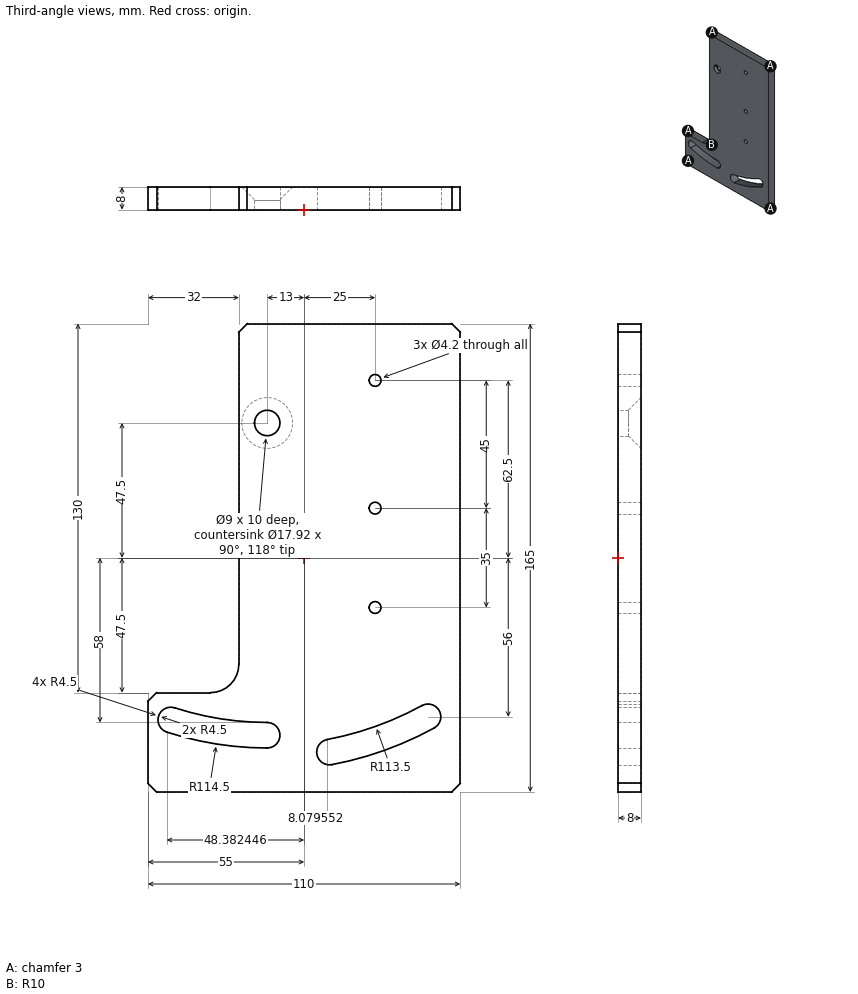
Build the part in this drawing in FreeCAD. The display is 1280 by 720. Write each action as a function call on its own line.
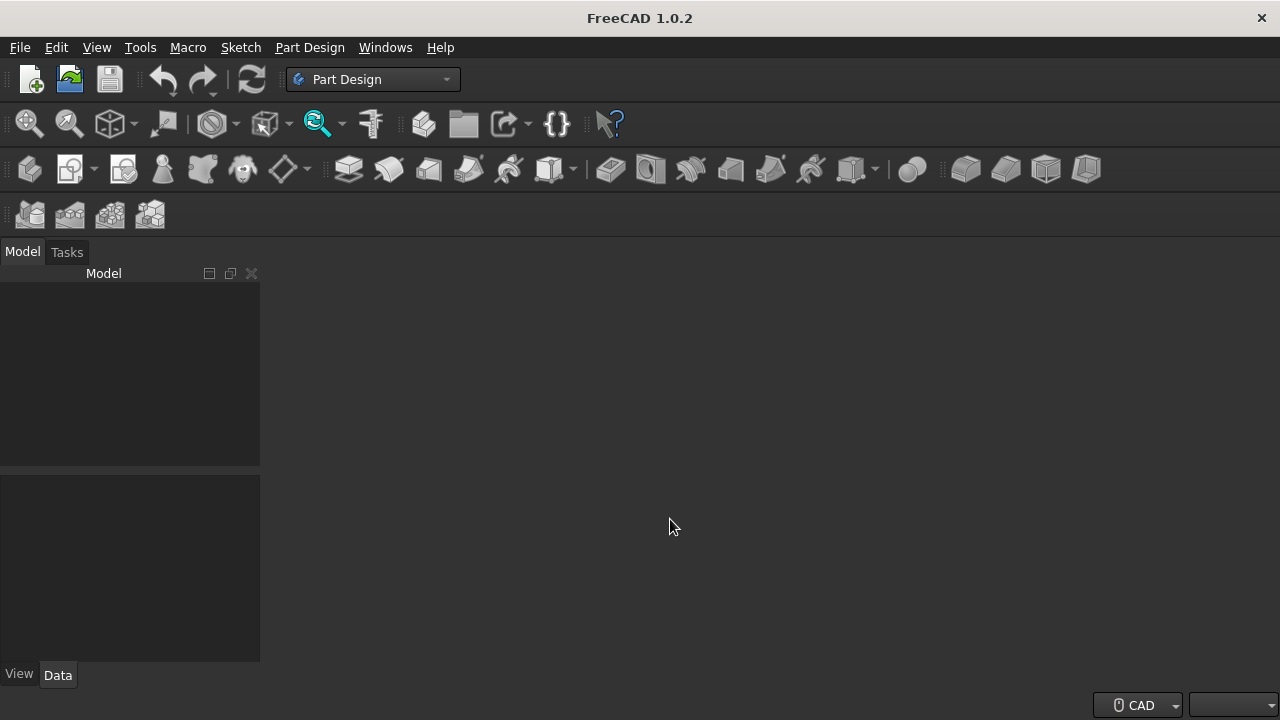
click(30, 80)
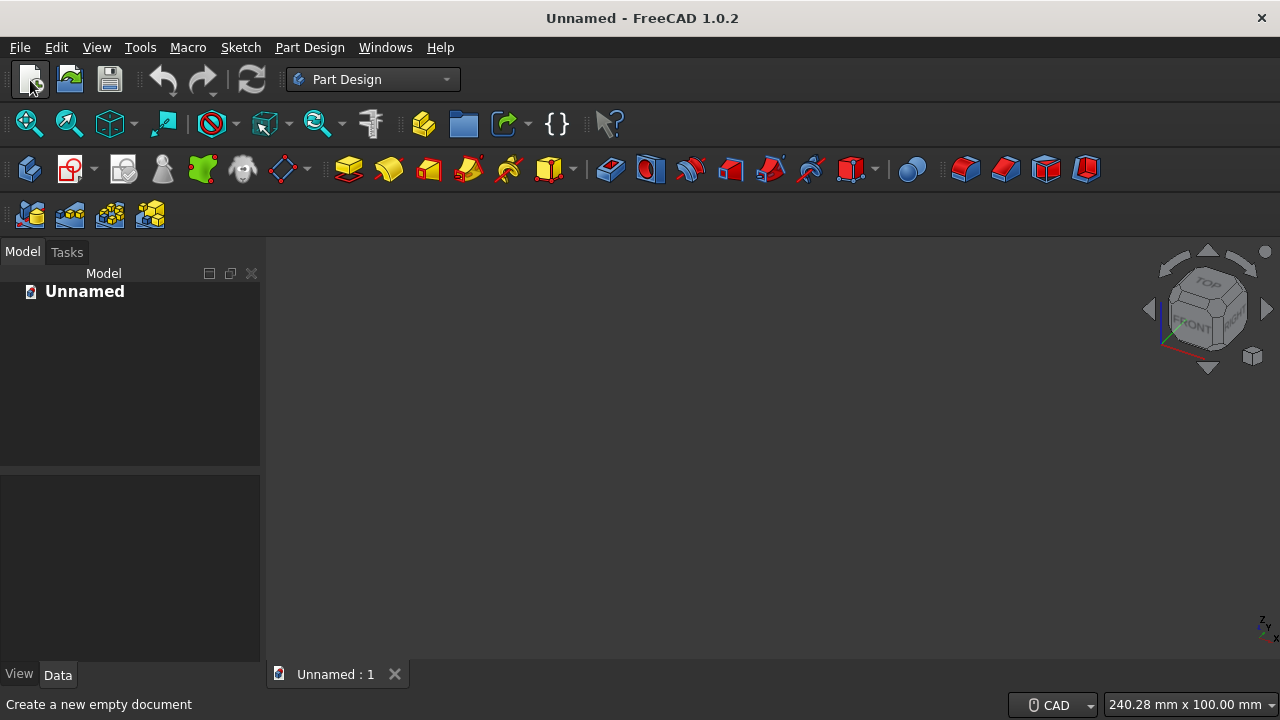
click(70, 170)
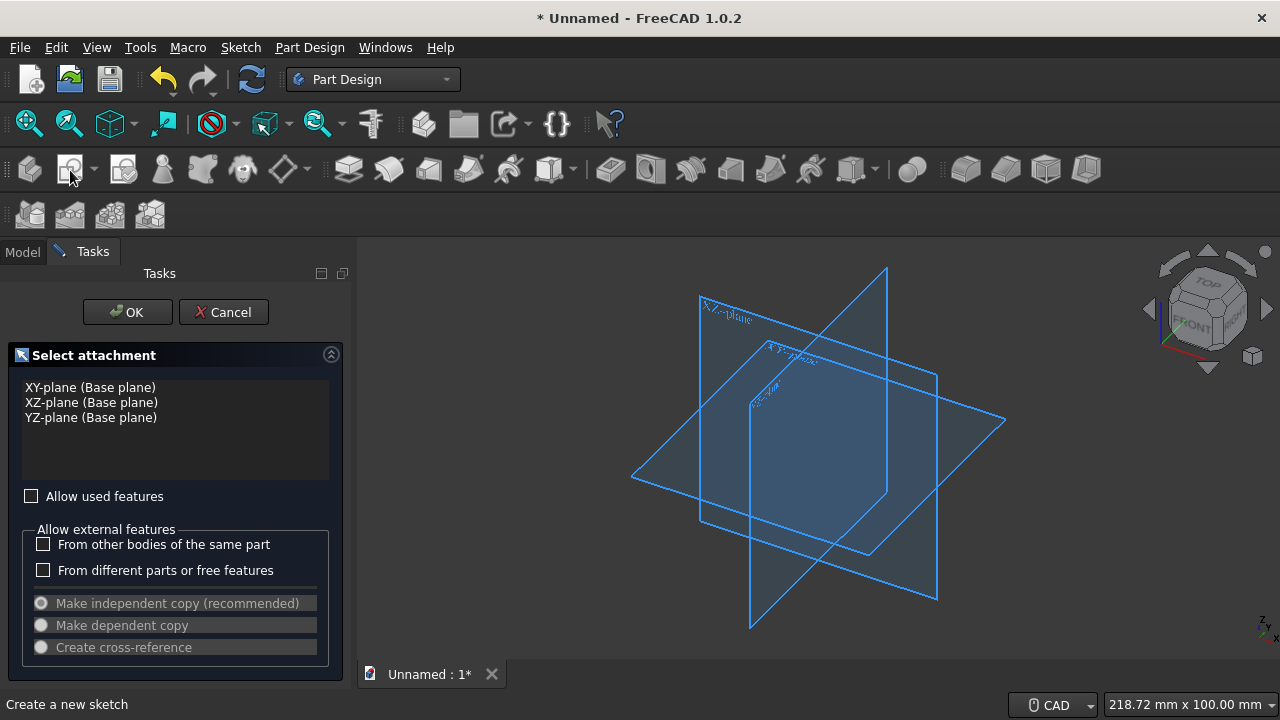
click(82, 402)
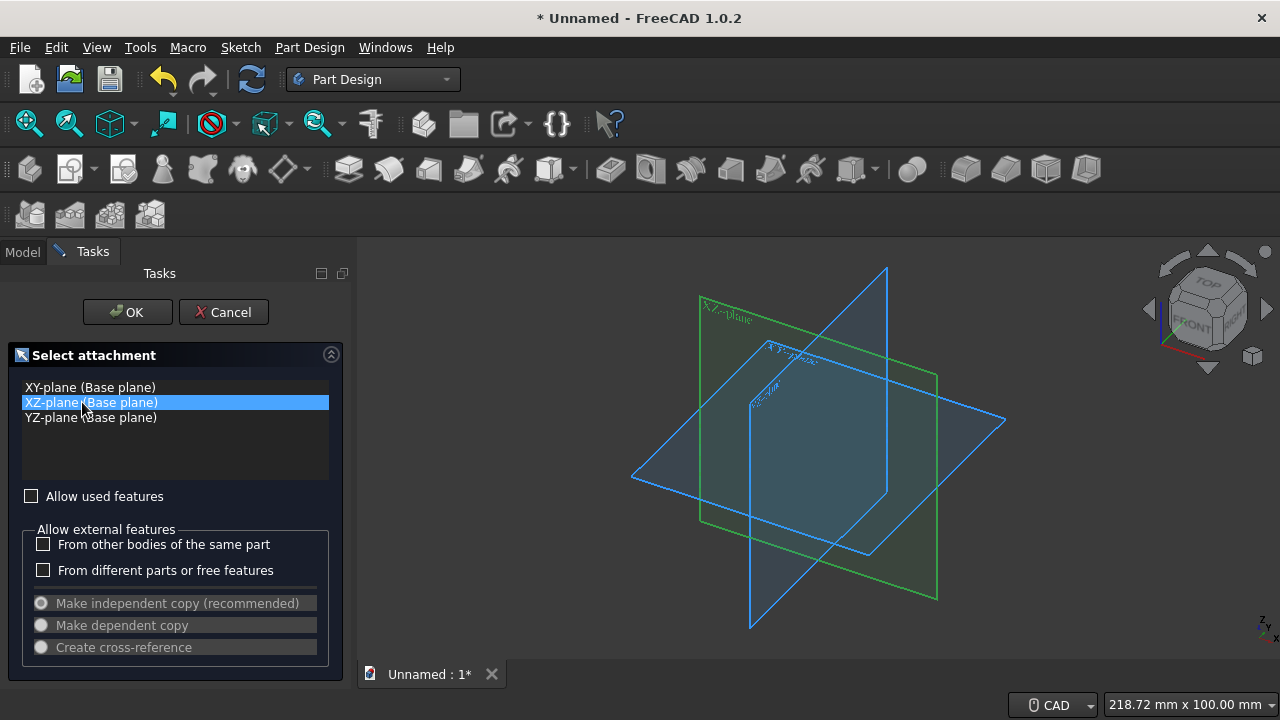
click(128, 312)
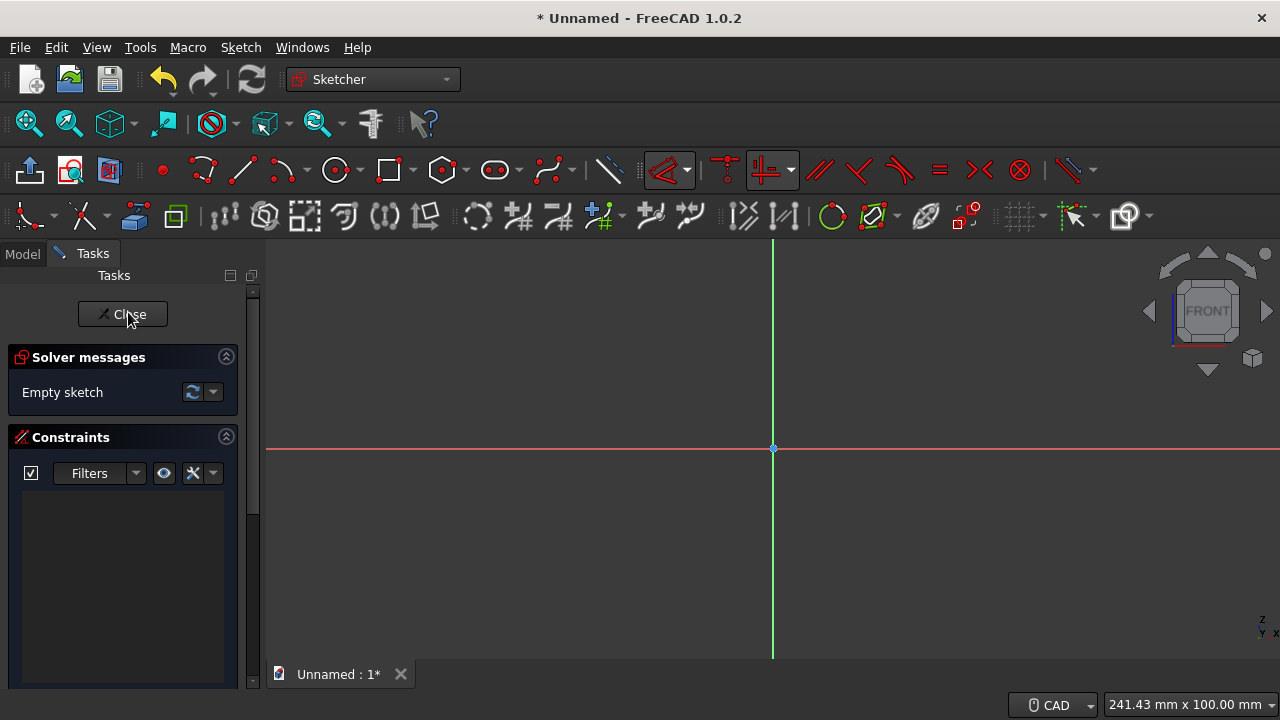
scroll(665, 449, down, 5)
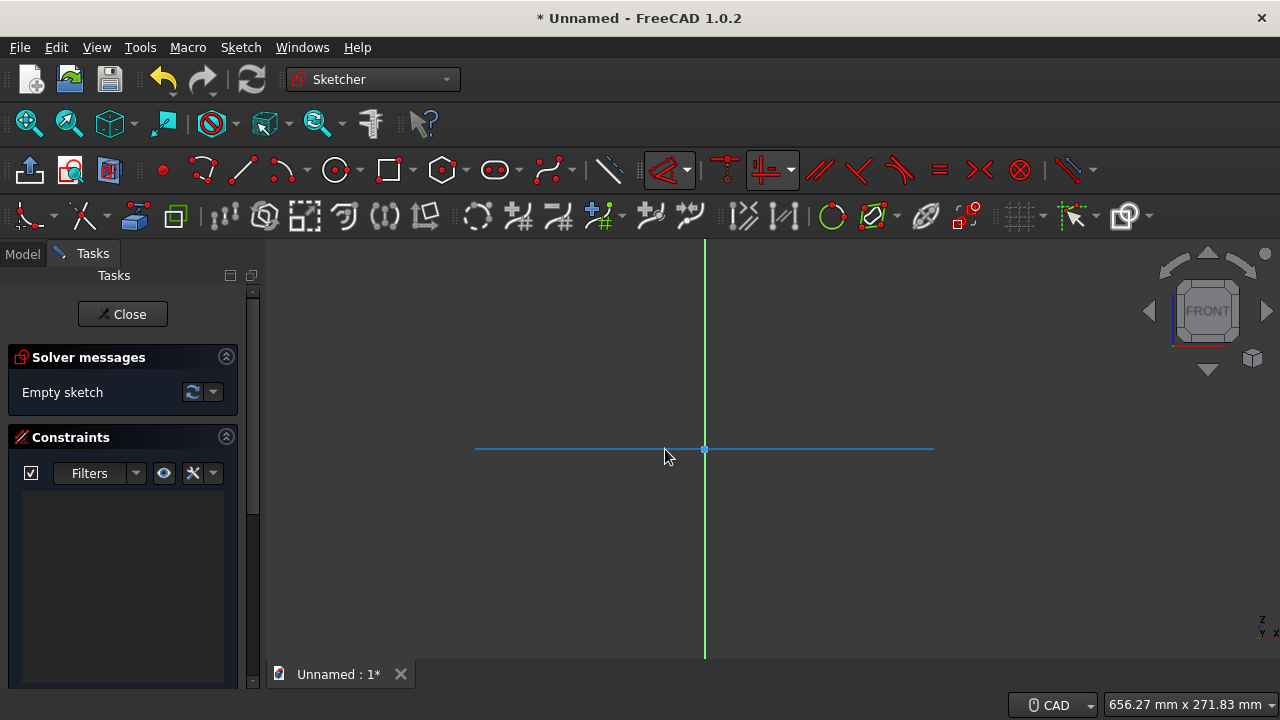
key(g)
key(v)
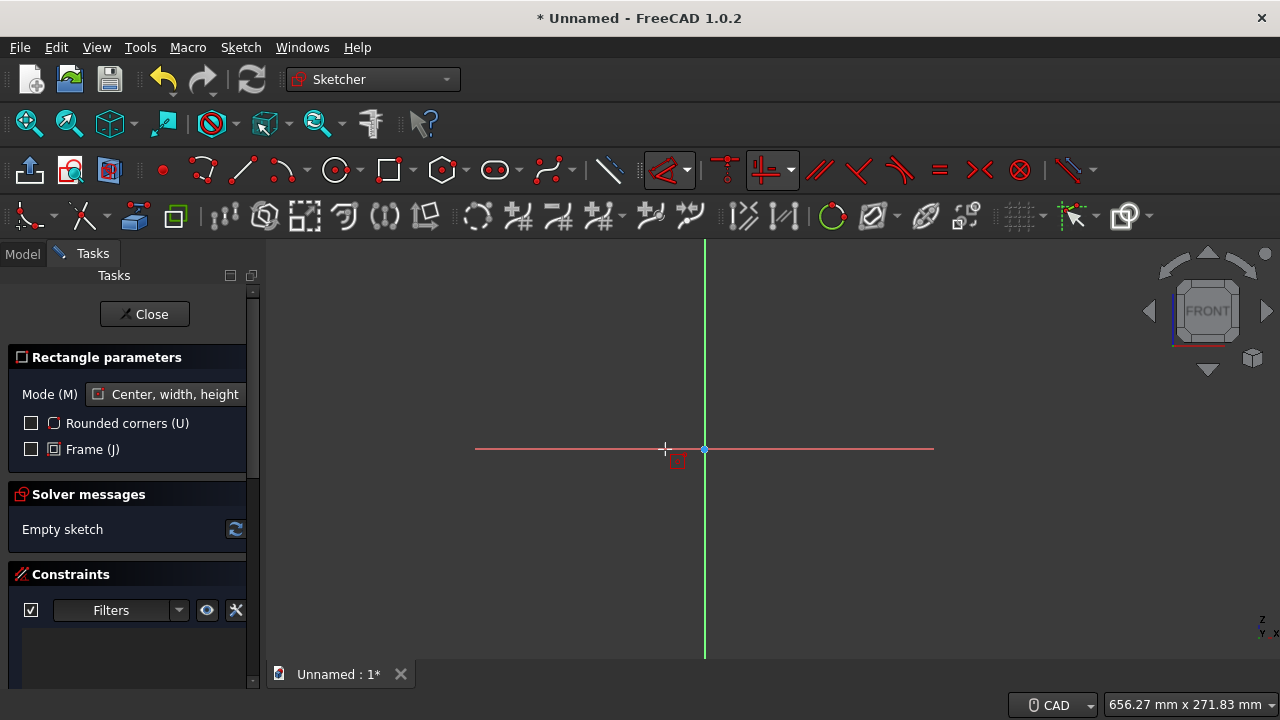
click(705, 449)
click(790, 322)
key(Escape)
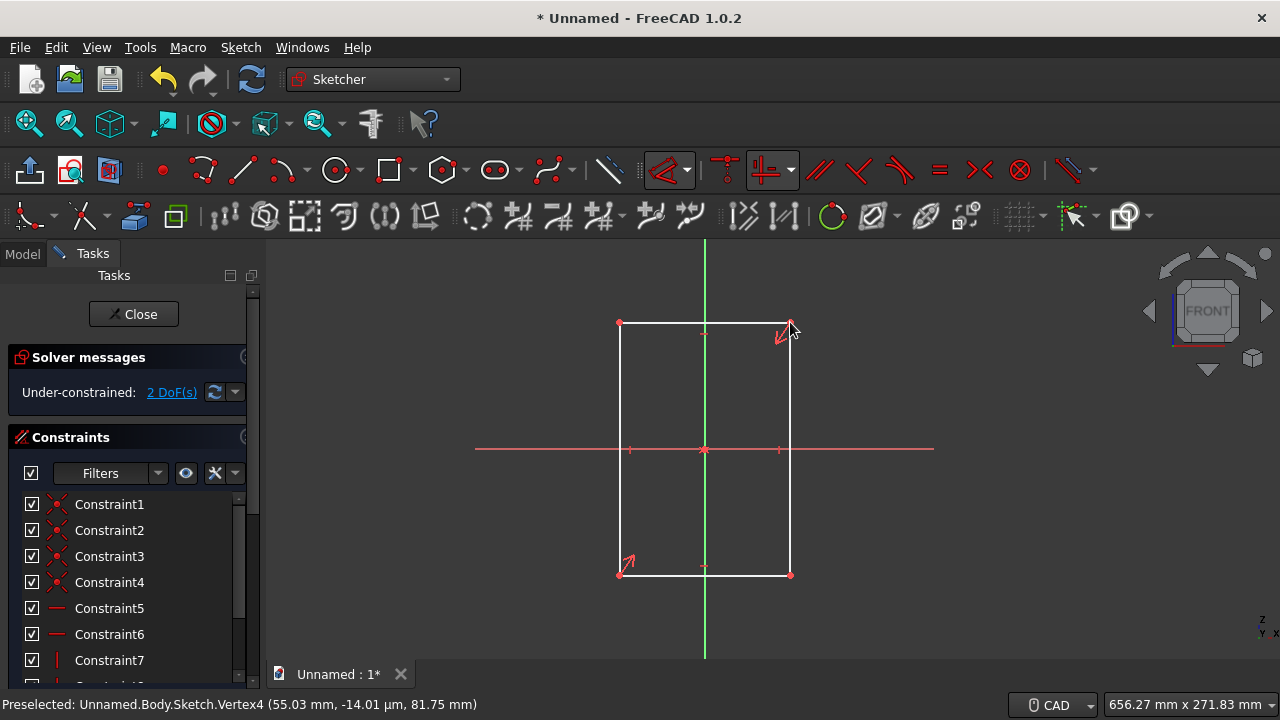
click(664, 170)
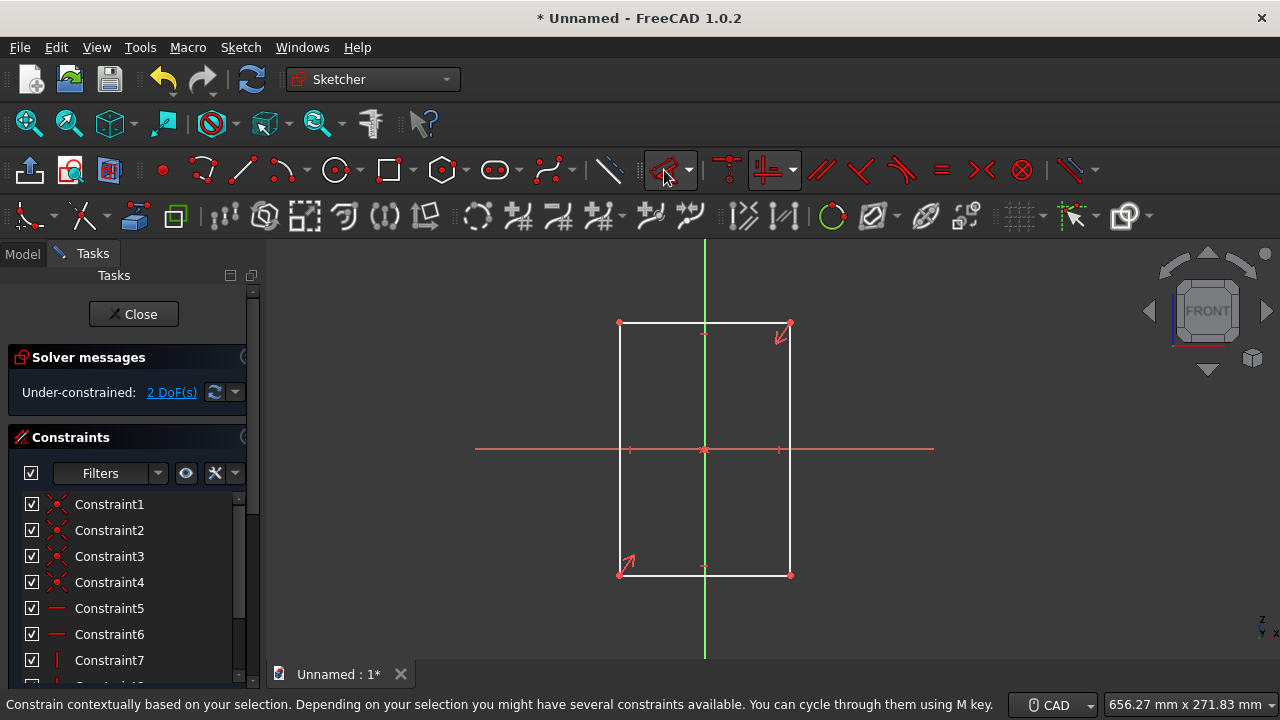
click(671, 576)
click(666, 610)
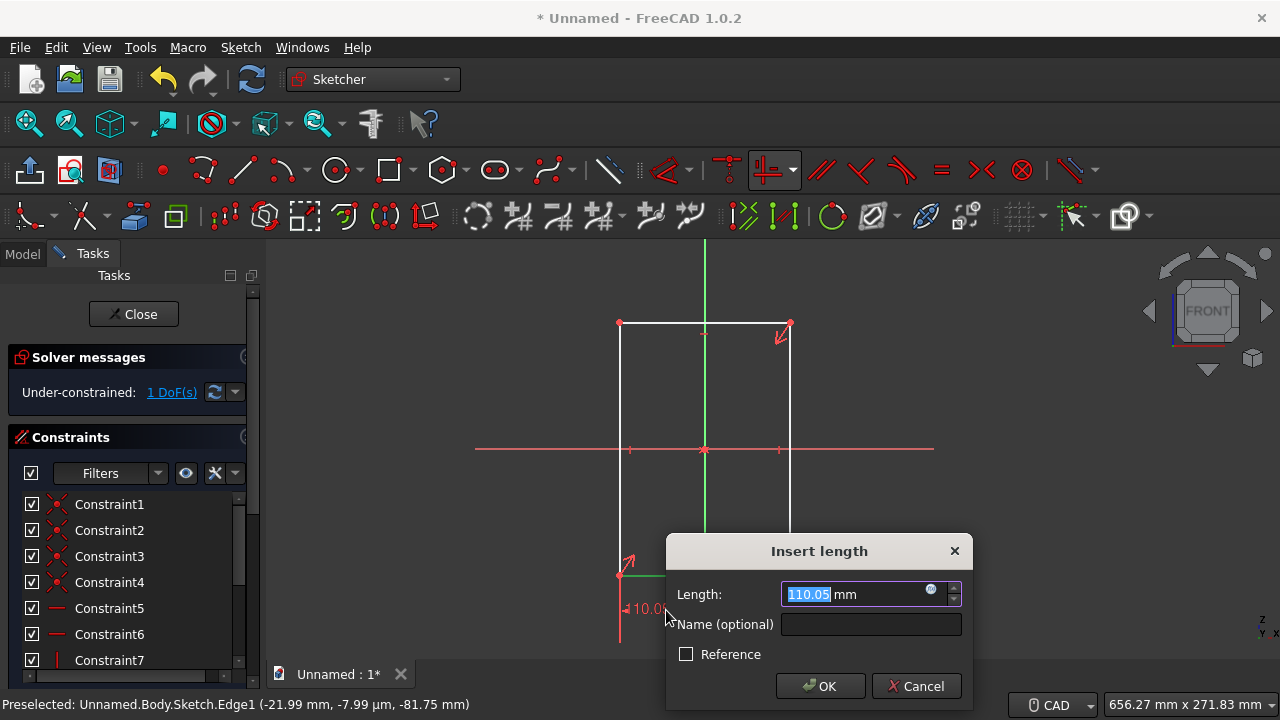
text(110)
key(Return)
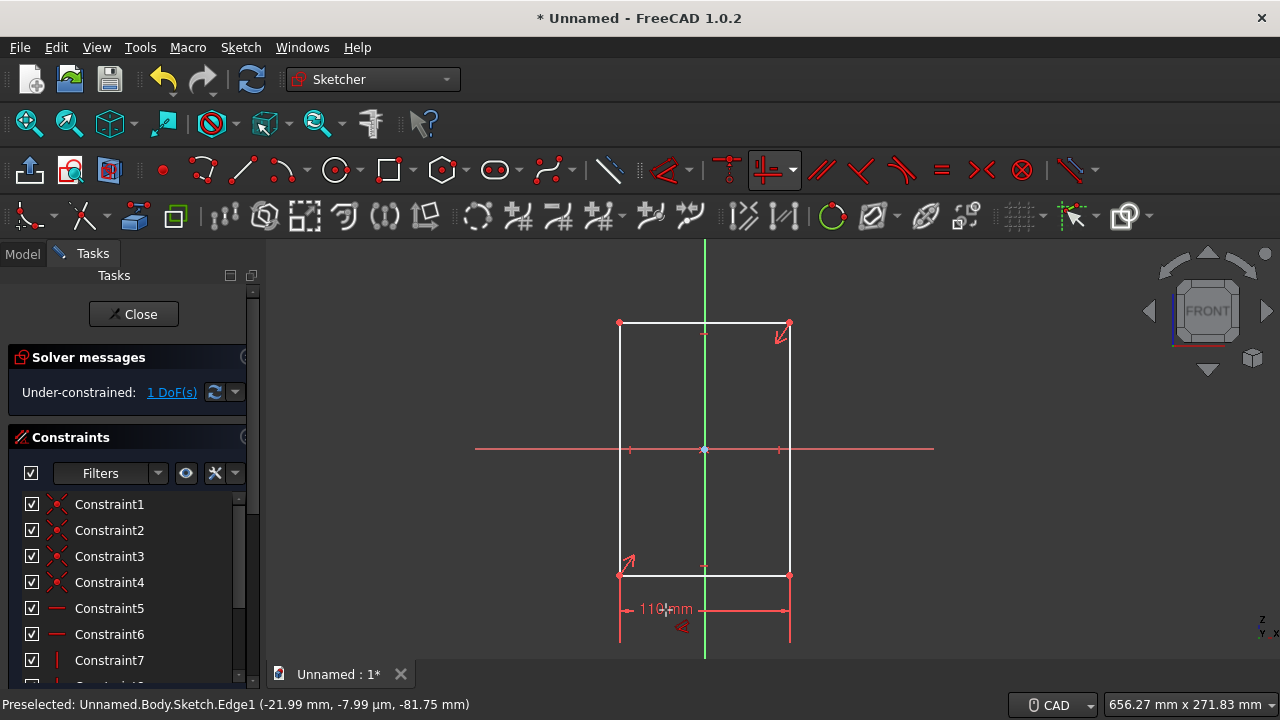
click(790, 500)
click(824, 391)